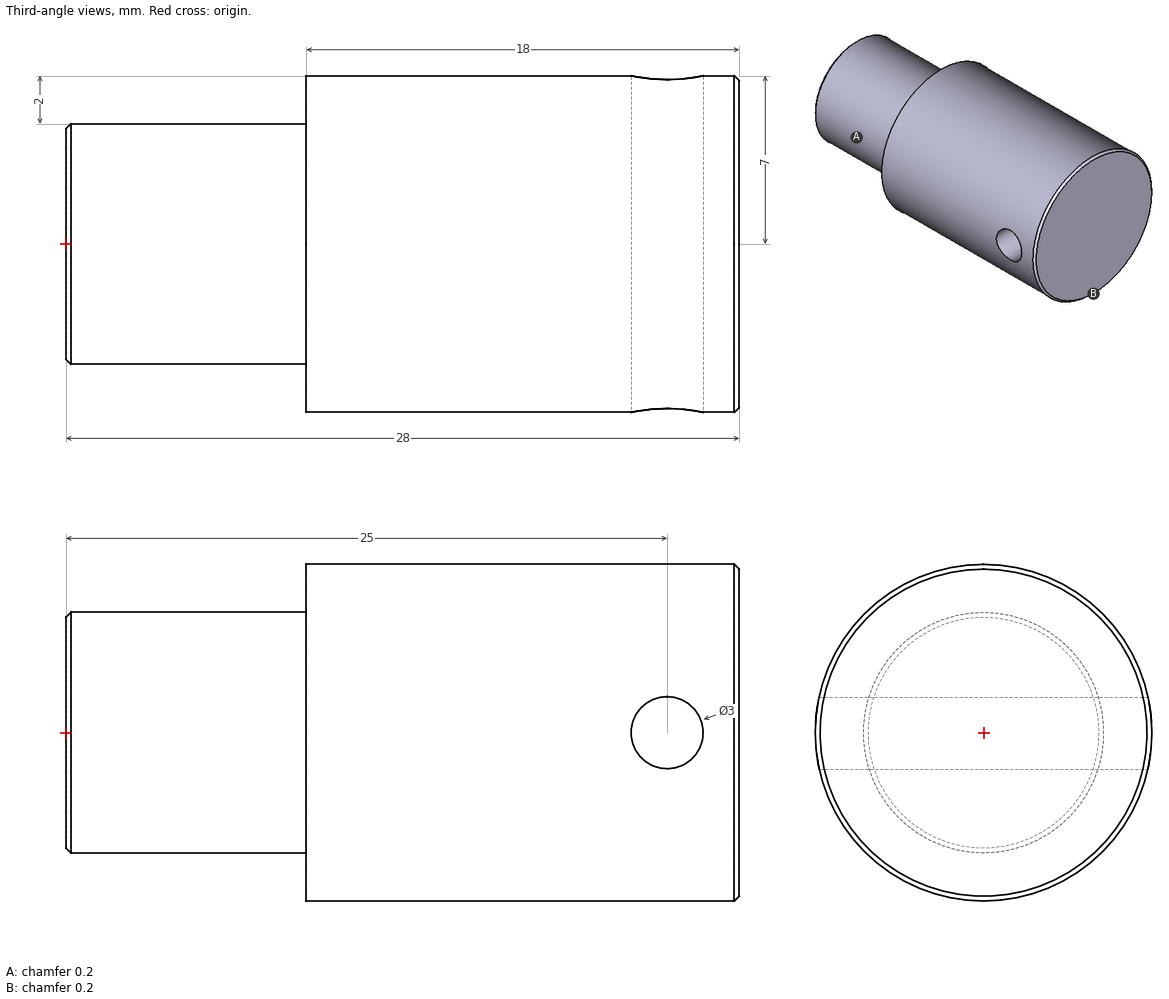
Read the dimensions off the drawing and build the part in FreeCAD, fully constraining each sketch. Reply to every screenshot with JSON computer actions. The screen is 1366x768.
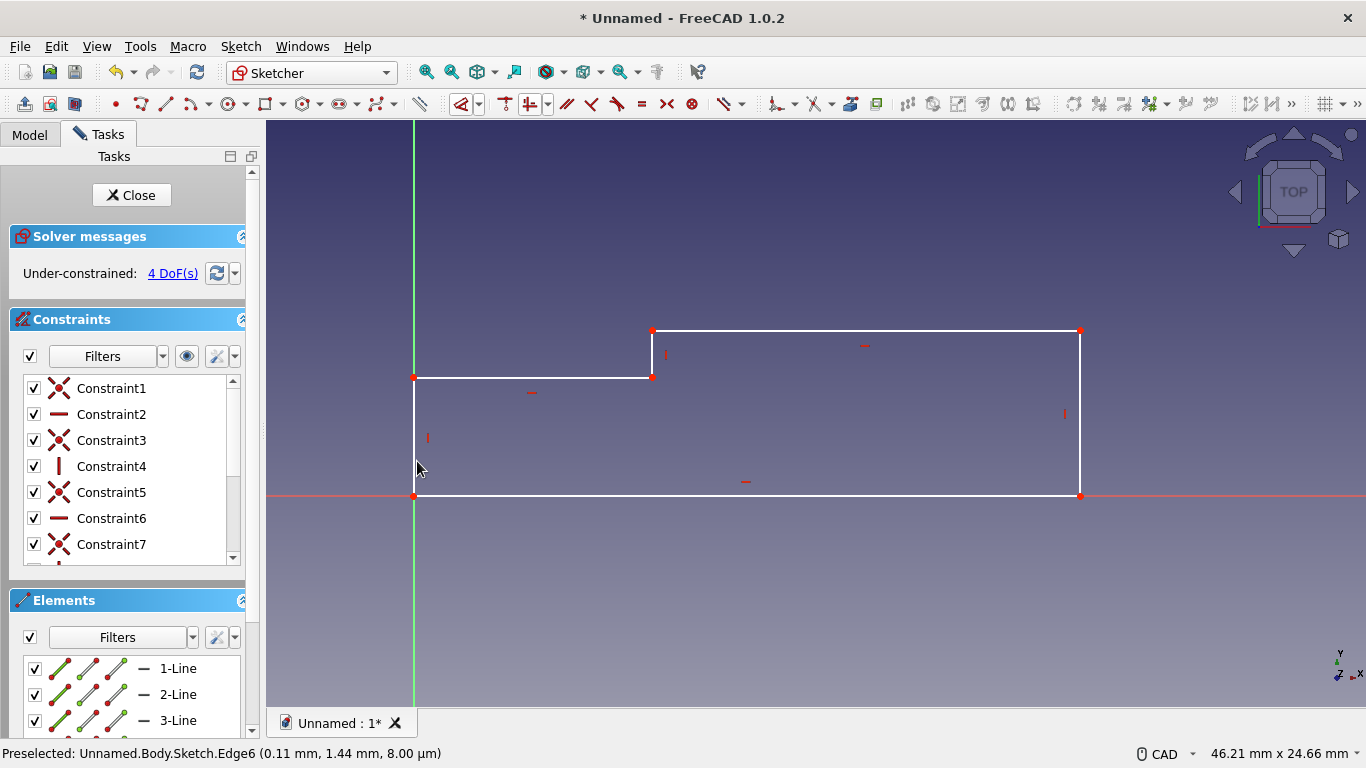
{"action": "key", "text": "d"}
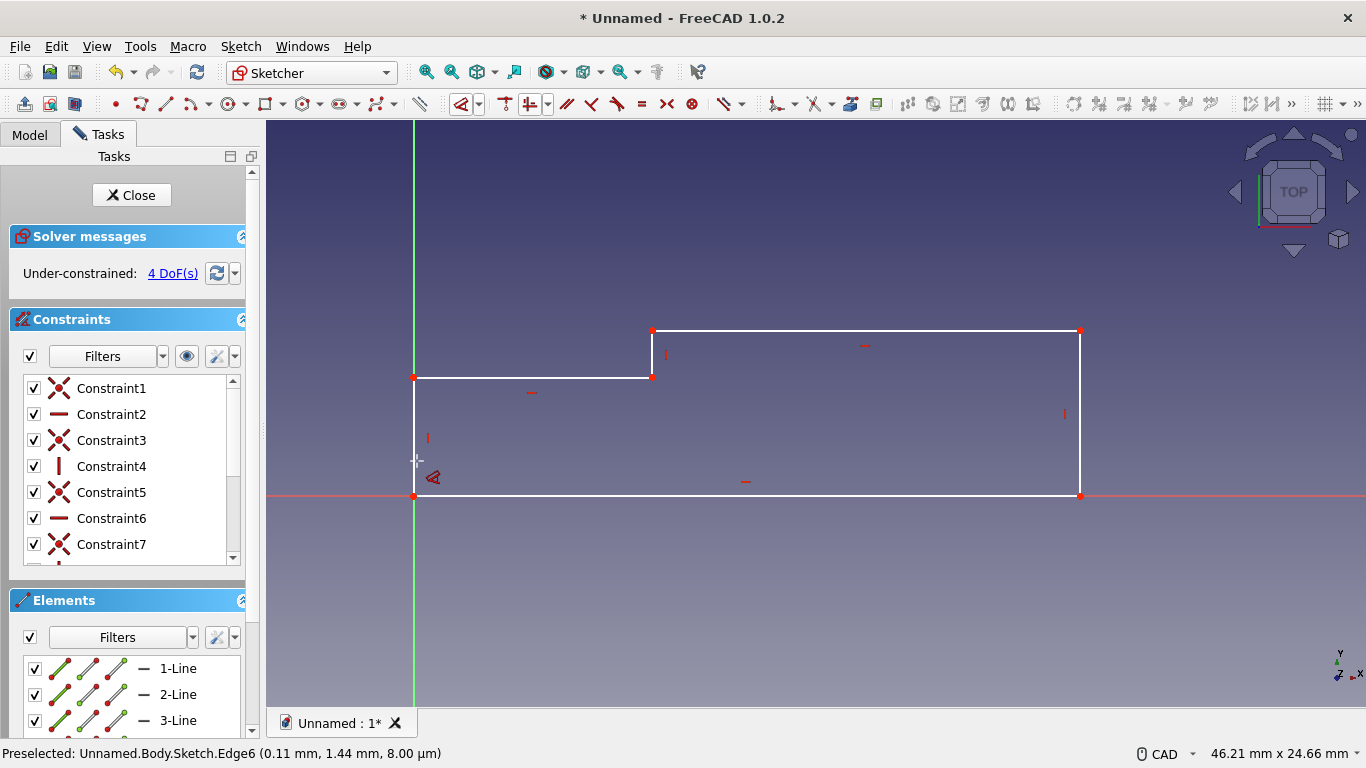
{"action": "left_click", "coordinate": [1080, 447]}
{"action": "left_click", "coordinate": [1114, 414]}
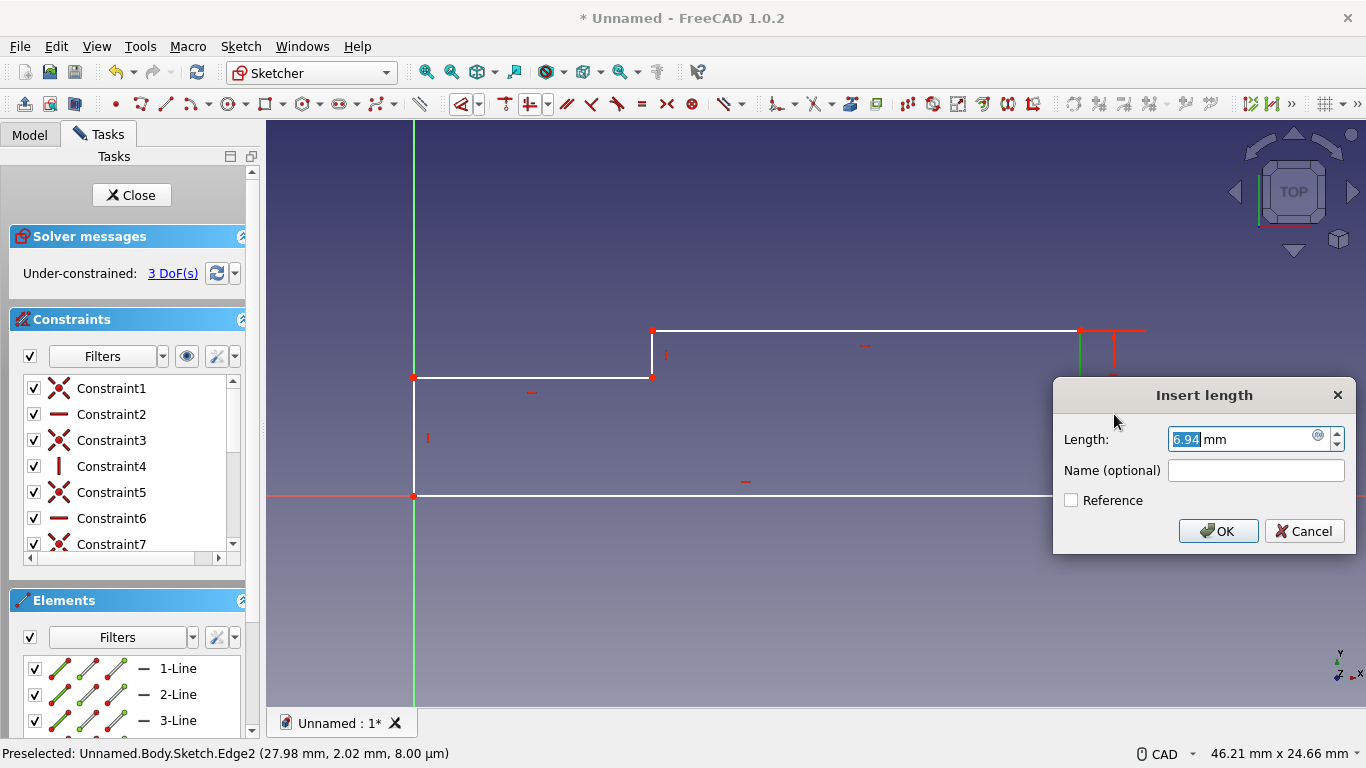
{"action": "type", "text": "7"}
{"action": "key", "text": "Return"}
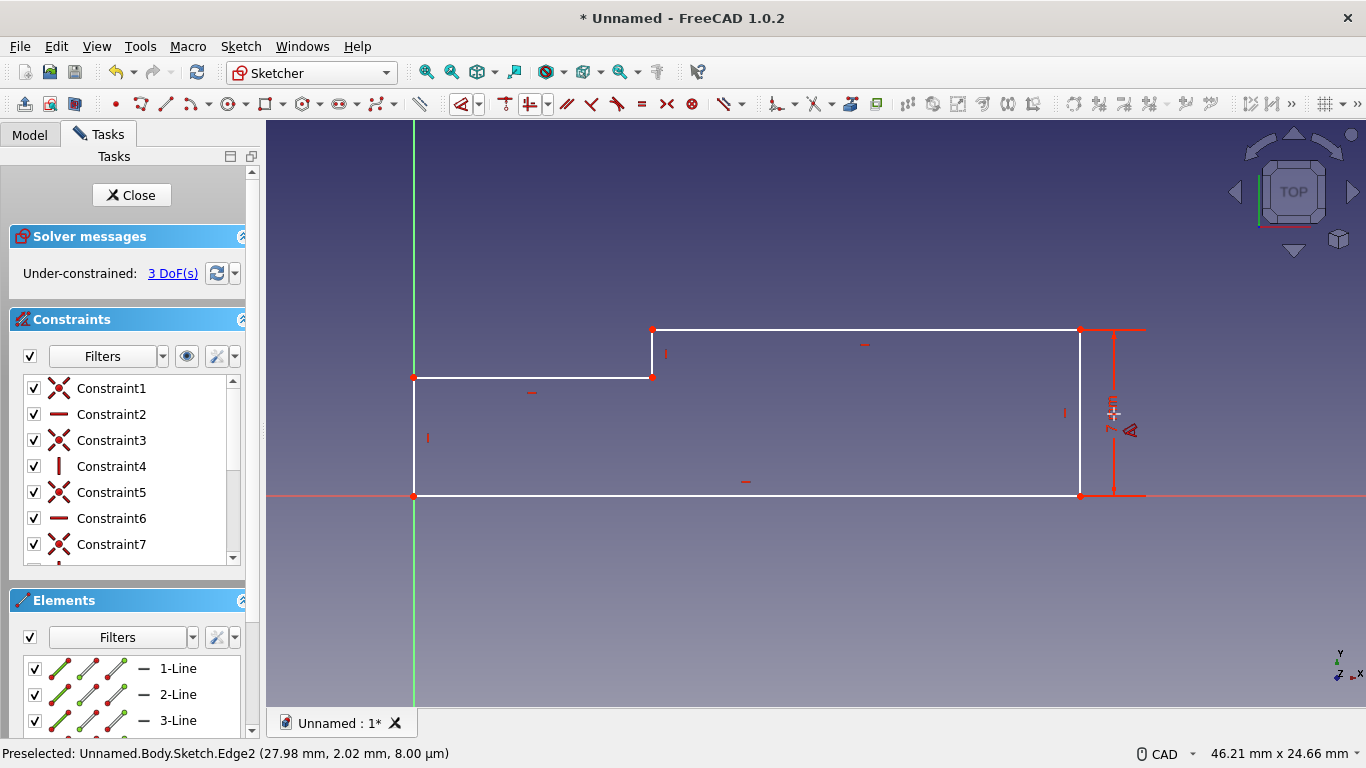
{"action": "left_click", "coordinate": [652, 344]}
{"action": "left_click", "coordinate": [618, 354]}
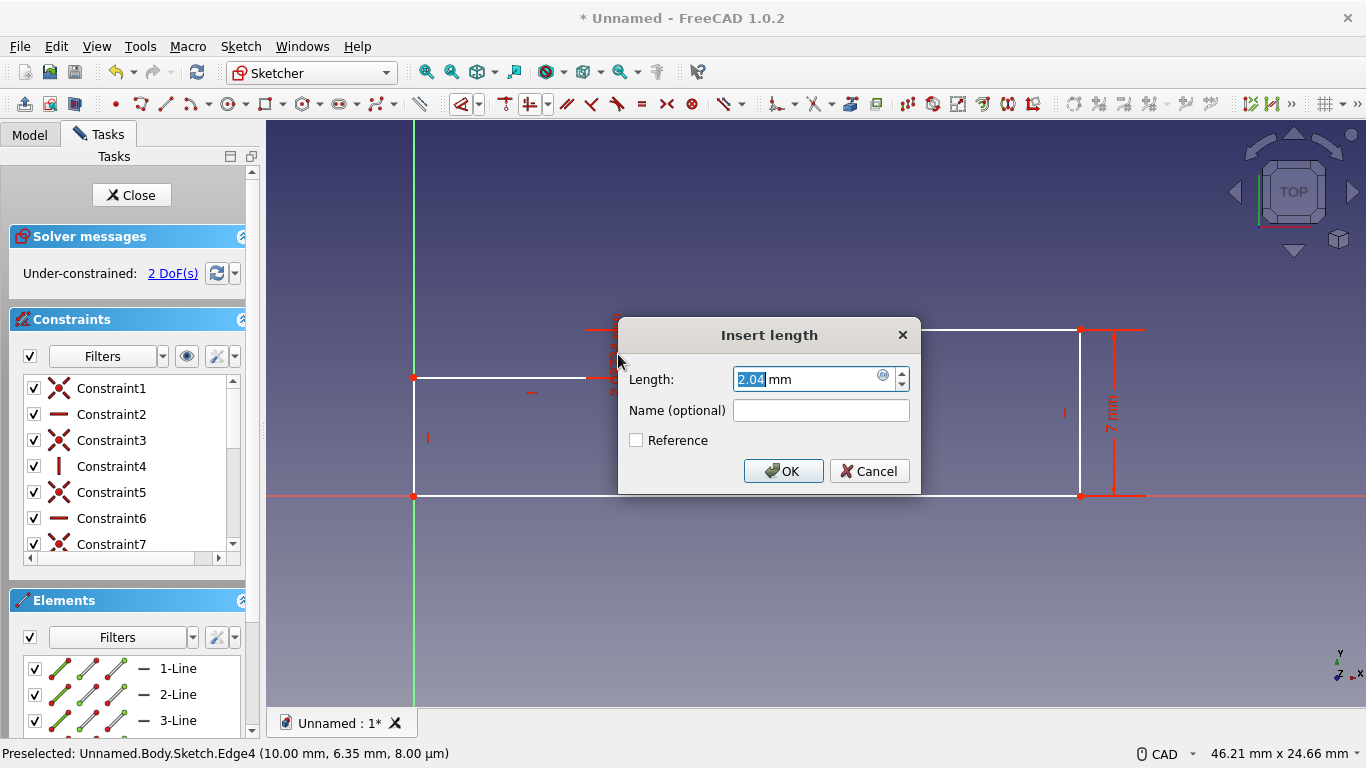
{"action": "type", "text": "2"}
{"action": "key", "text": "Return"}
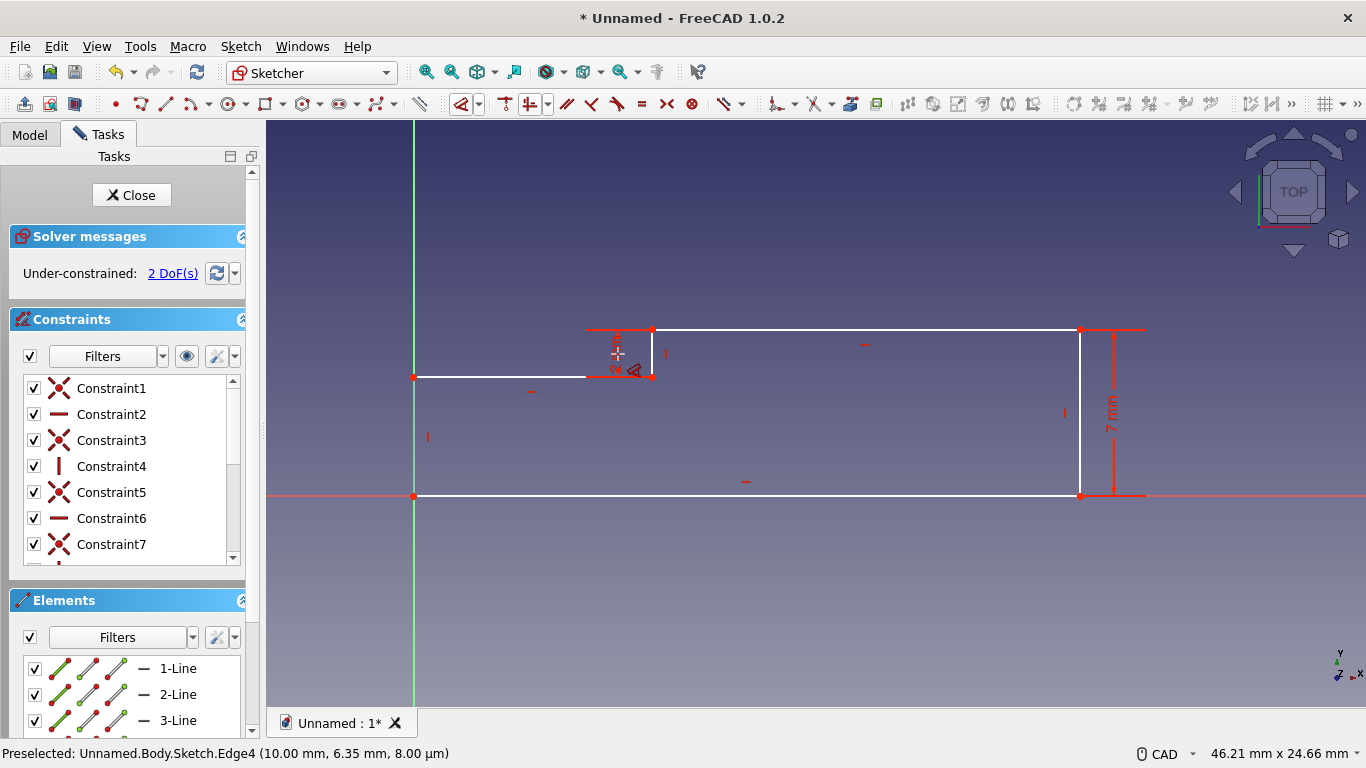
{"action": "left_click", "coordinate": [614, 496]}
{"action": "left_click", "coordinate": [747, 530]}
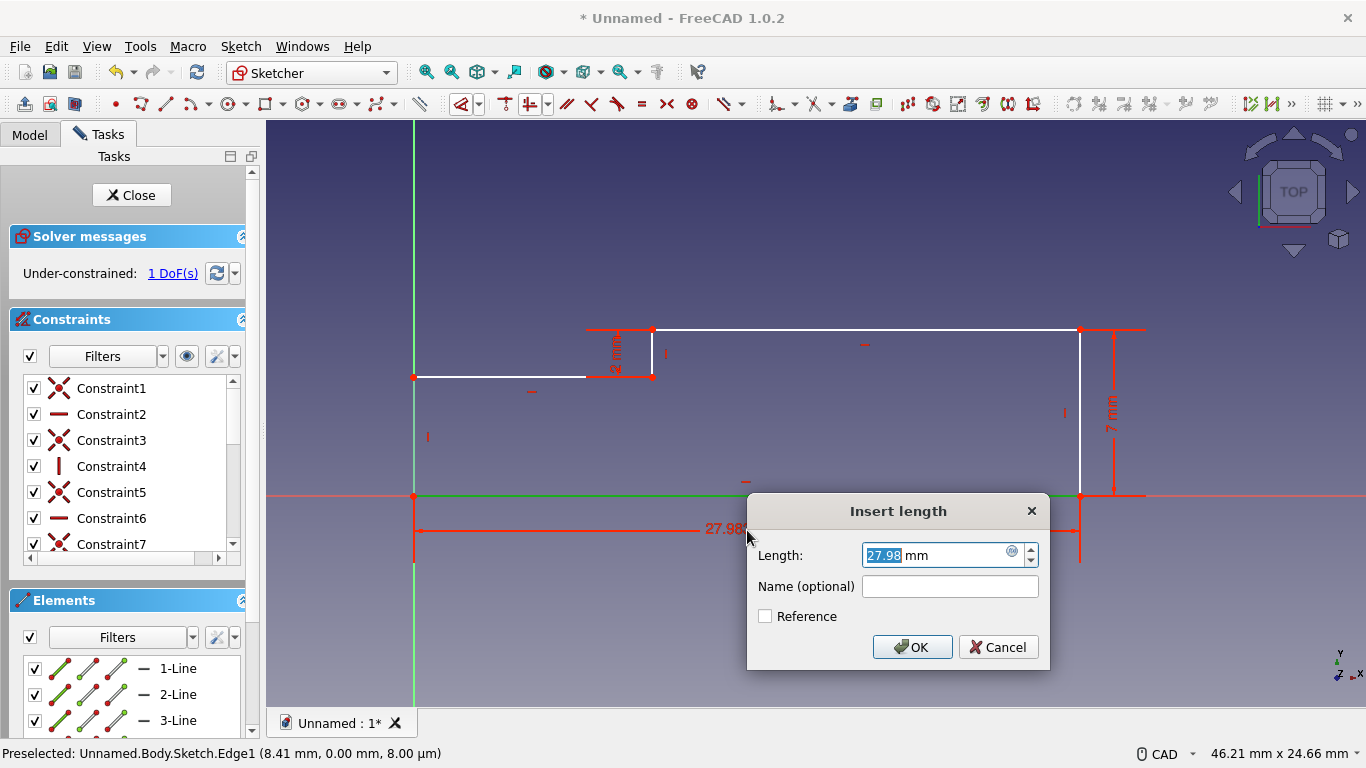
{"action": "type", "text": "28"}
{"action": "key", "text": "Return"}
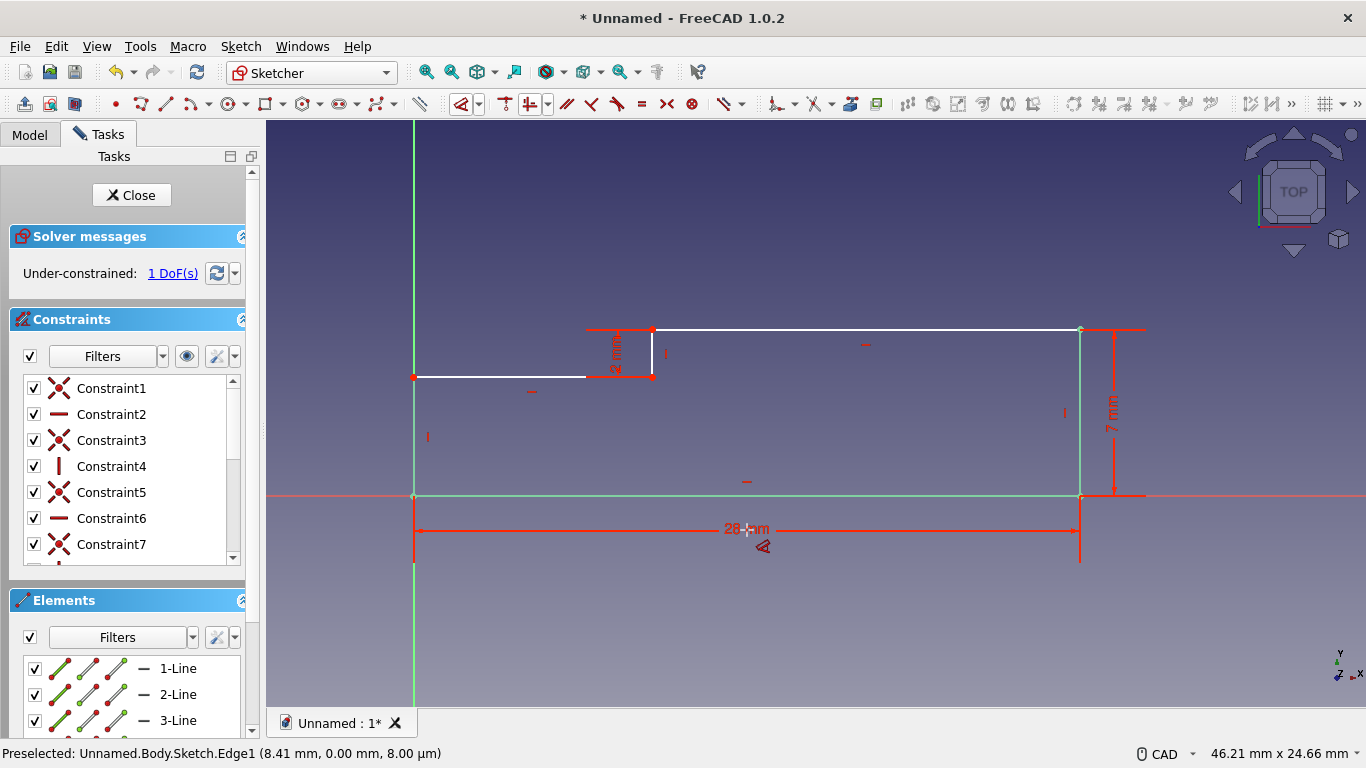
{"action": "left_click", "coordinate": [952, 330]}
{"action": "left_click", "coordinate": [866, 296]}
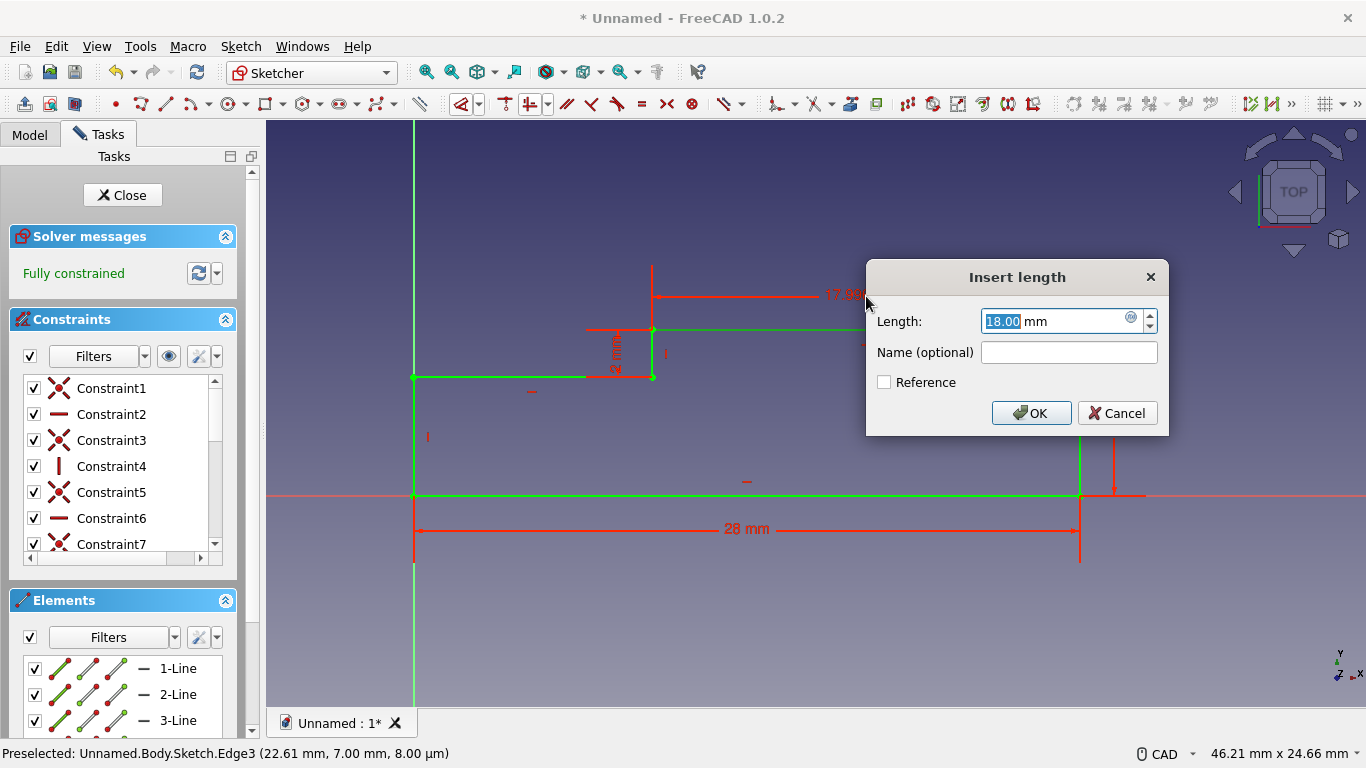
{"action": "type", "text": "18"}
{"action": "key", "text": "Return"}
{"action": "key", "text": "Escape"}